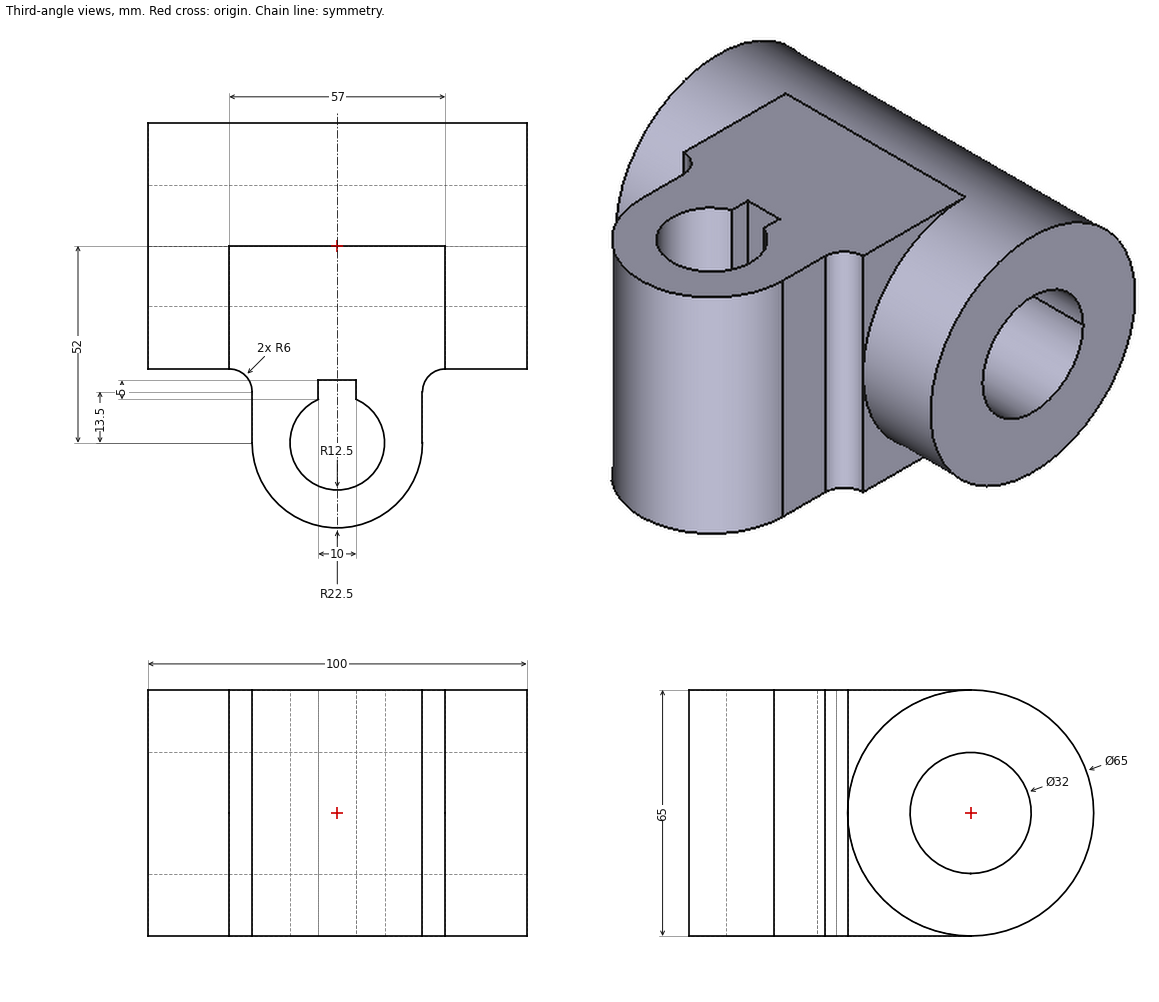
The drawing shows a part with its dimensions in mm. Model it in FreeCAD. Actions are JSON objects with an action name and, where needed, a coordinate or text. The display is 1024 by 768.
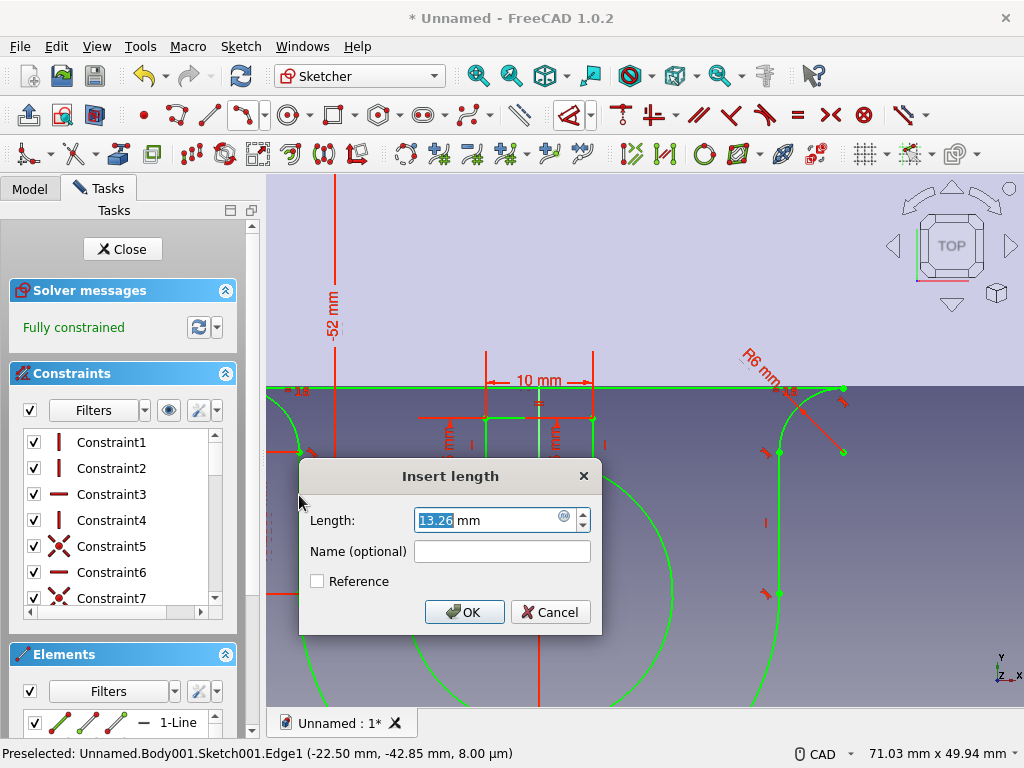
{"action": "type", "text": "13.5"}
{"action": "key", "text": "Return"}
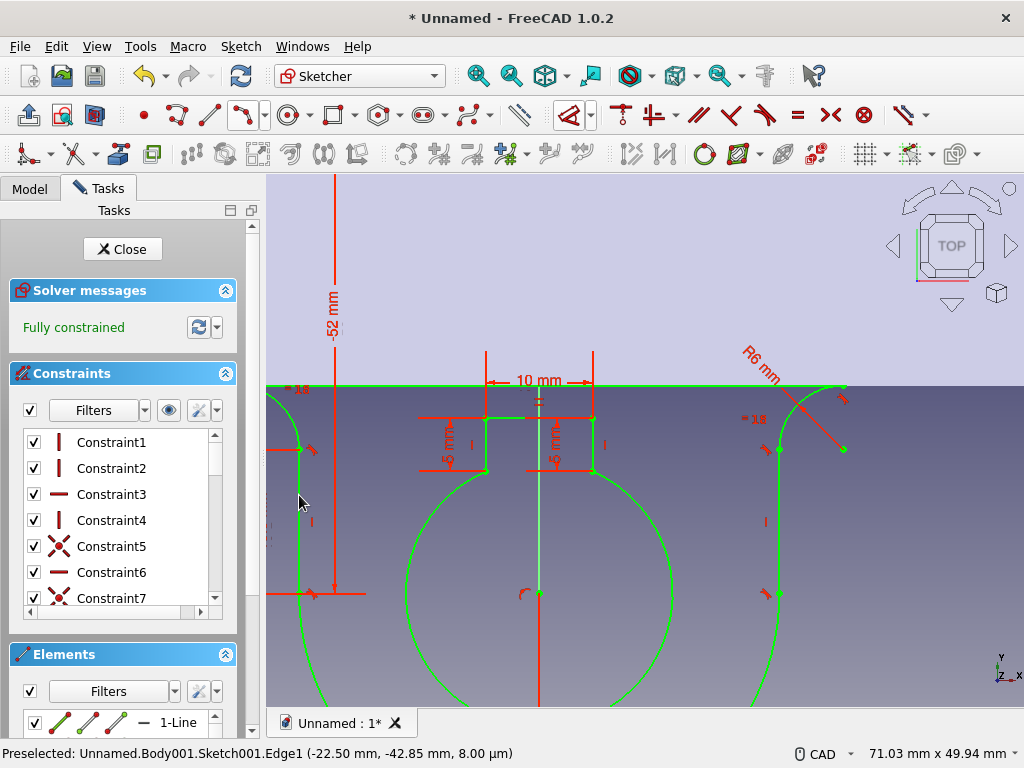
{"action": "left_click", "coordinate": [123, 249]}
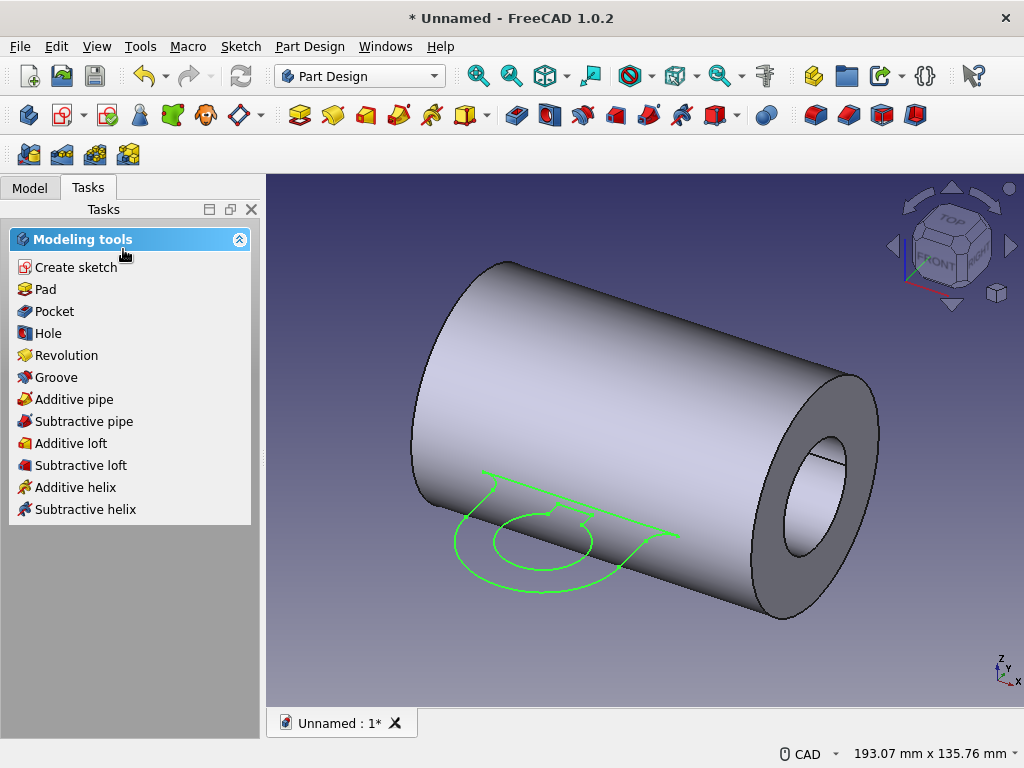
{"action": "left_click", "coordinate": [300, 116]}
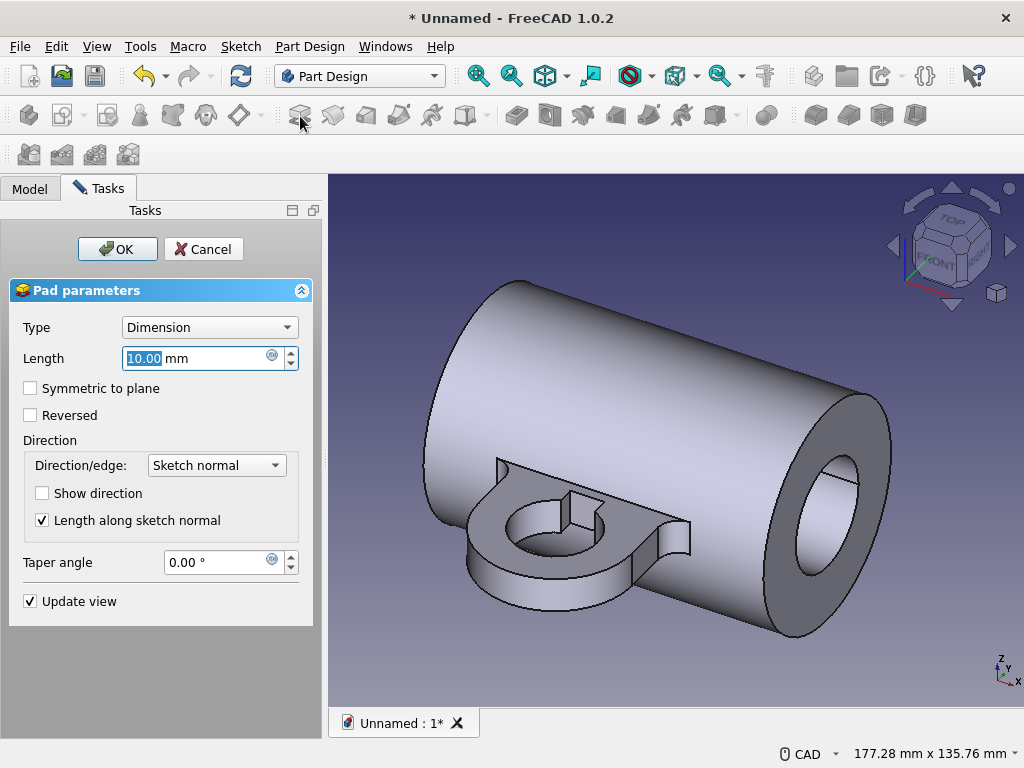
{"action": "type", "text": "65"}
{"action": "key", "text": "Tab"}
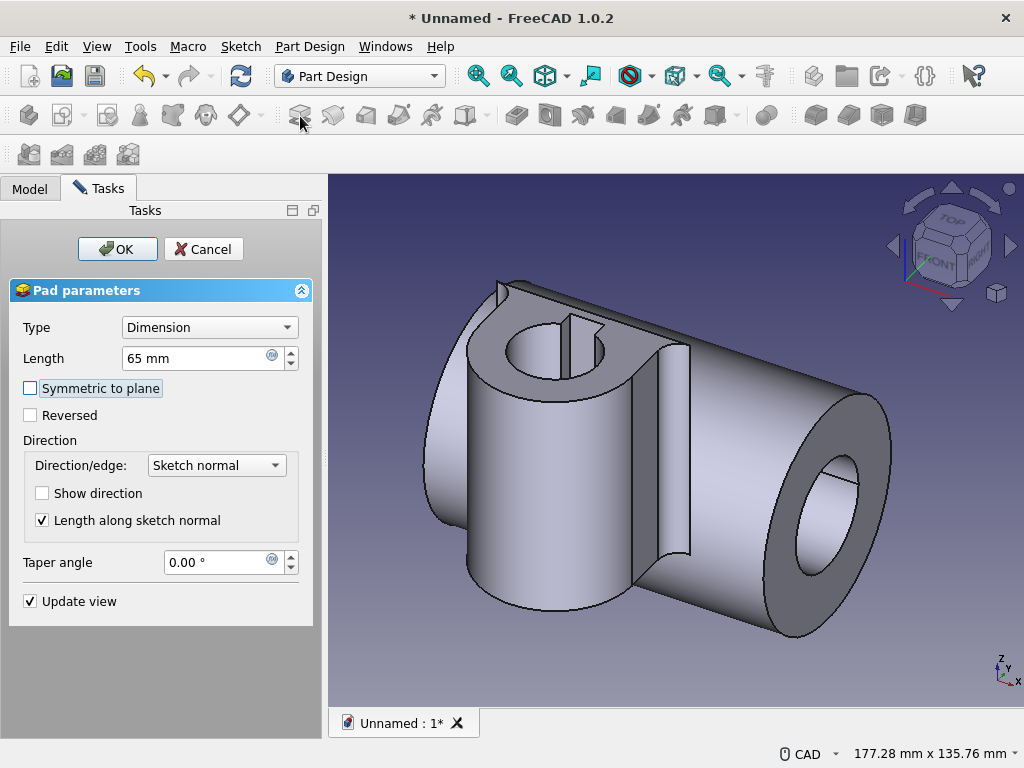
{"action": "left_click", "coordinate": [31, 388]}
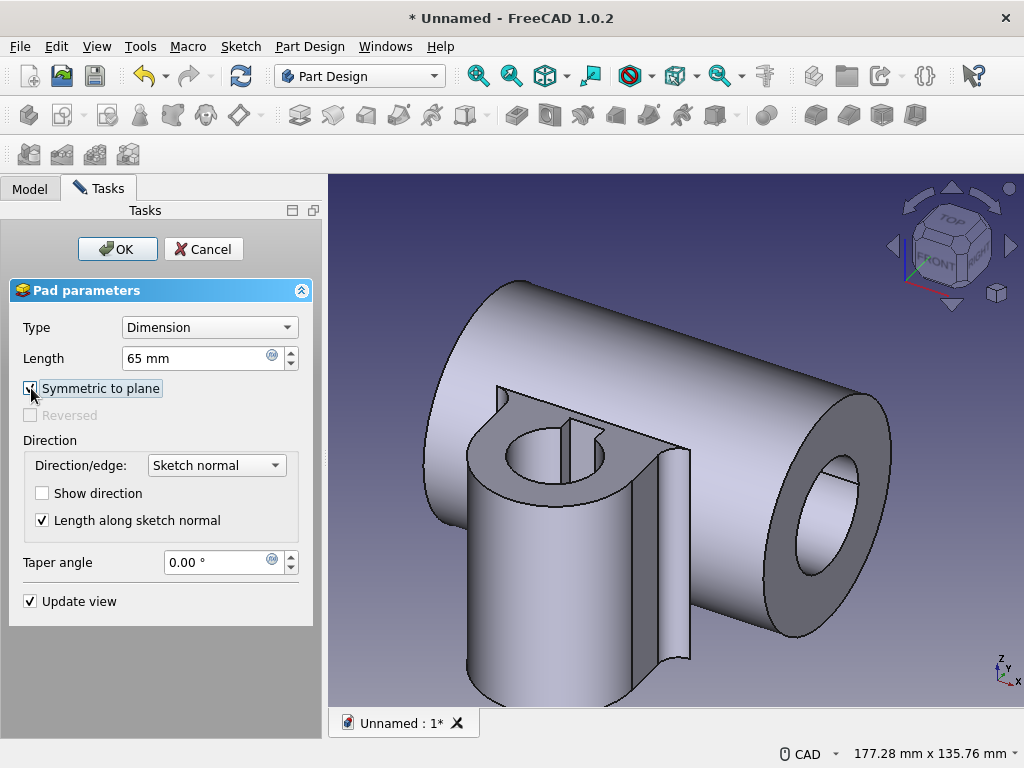
{"action": "left_click", "coordinate": [118, 249]}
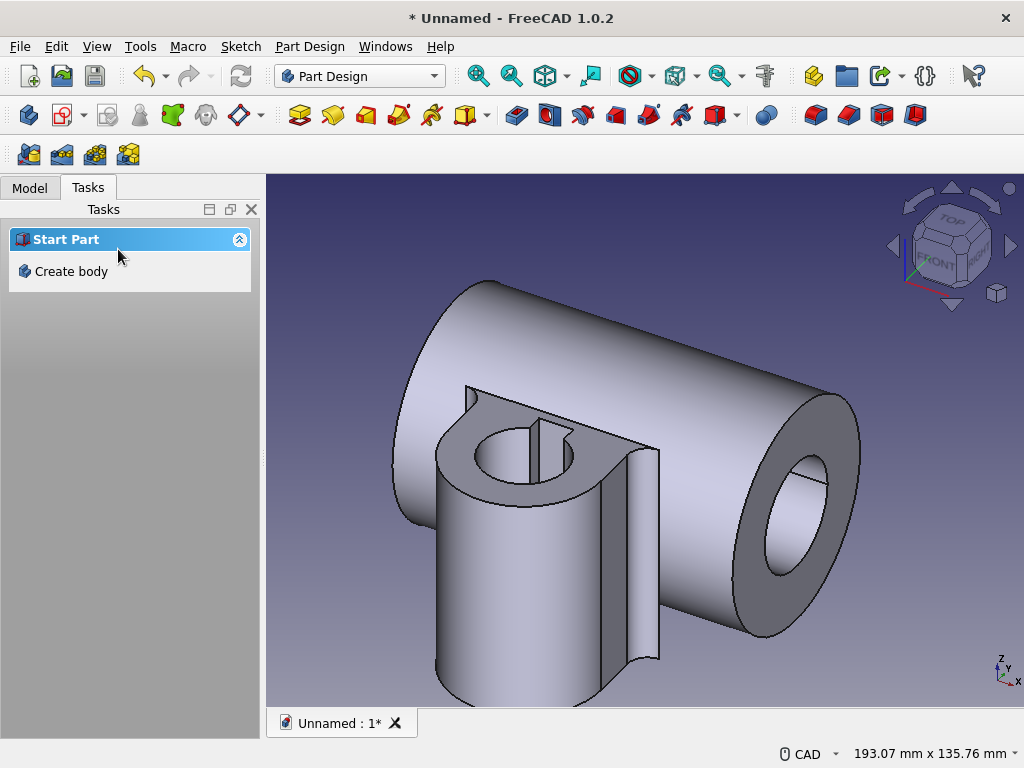
{"action": "key", "text": "v f"}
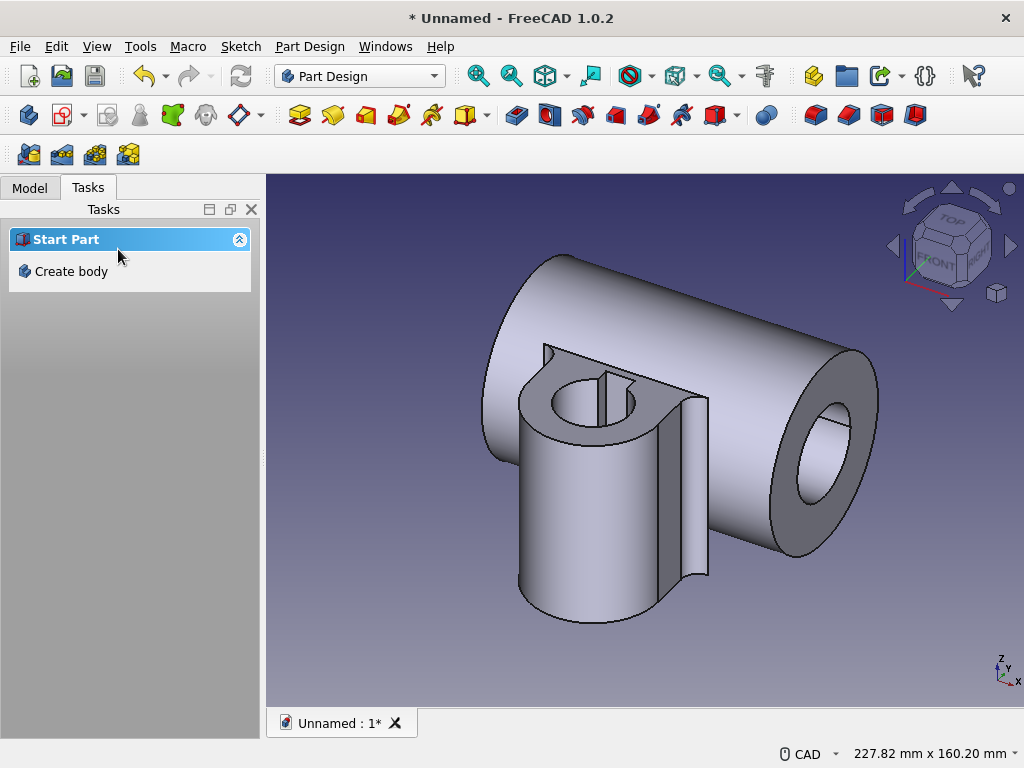
{"action": "left_click", "coordinate": [30, 188]}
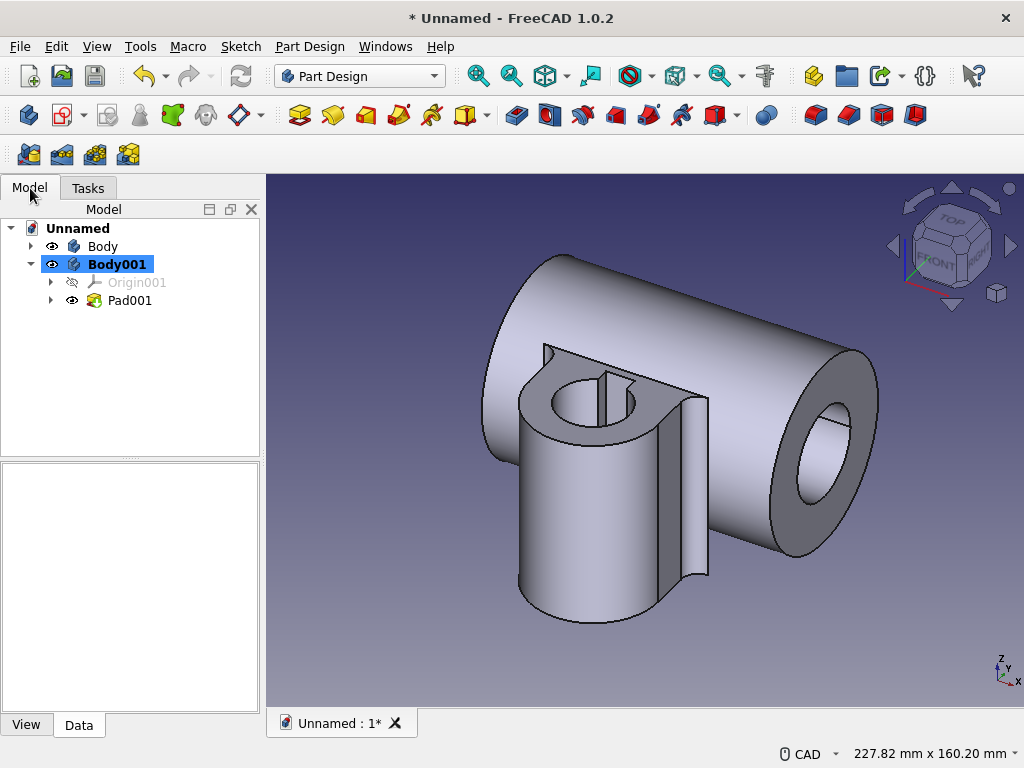
{"action": "double_click", "coordinate": [97, 246]}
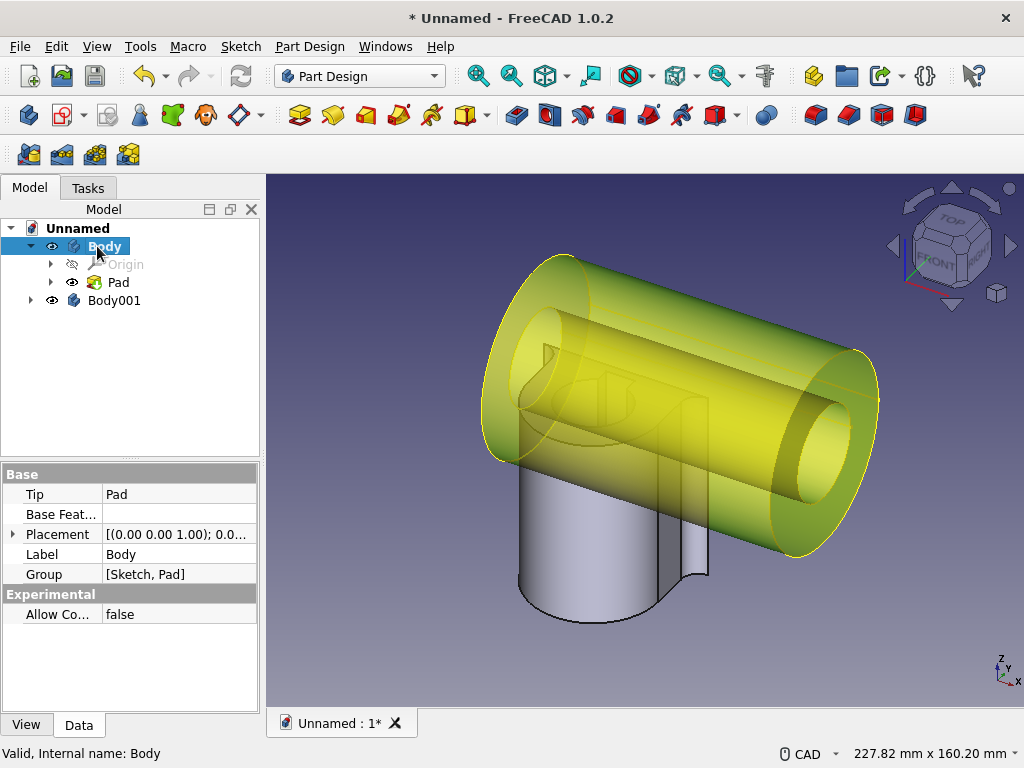
{"action": "left_click", "coordinate": [97, 246]}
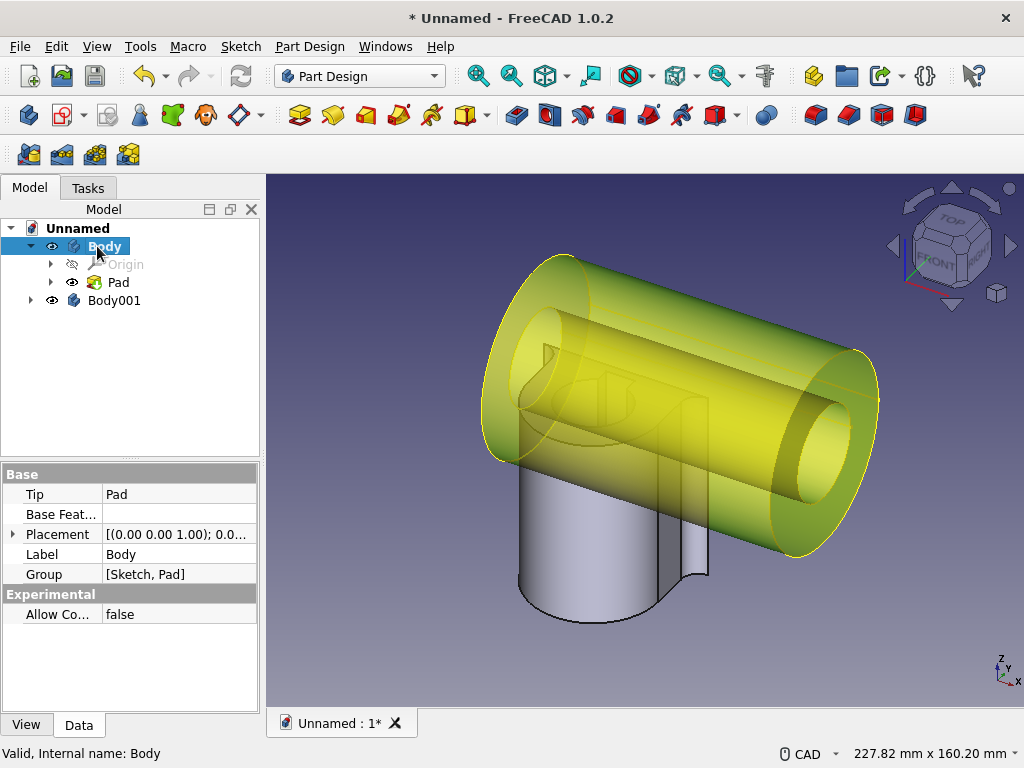
{"action": "left_click", "coordinate": [148, 614]}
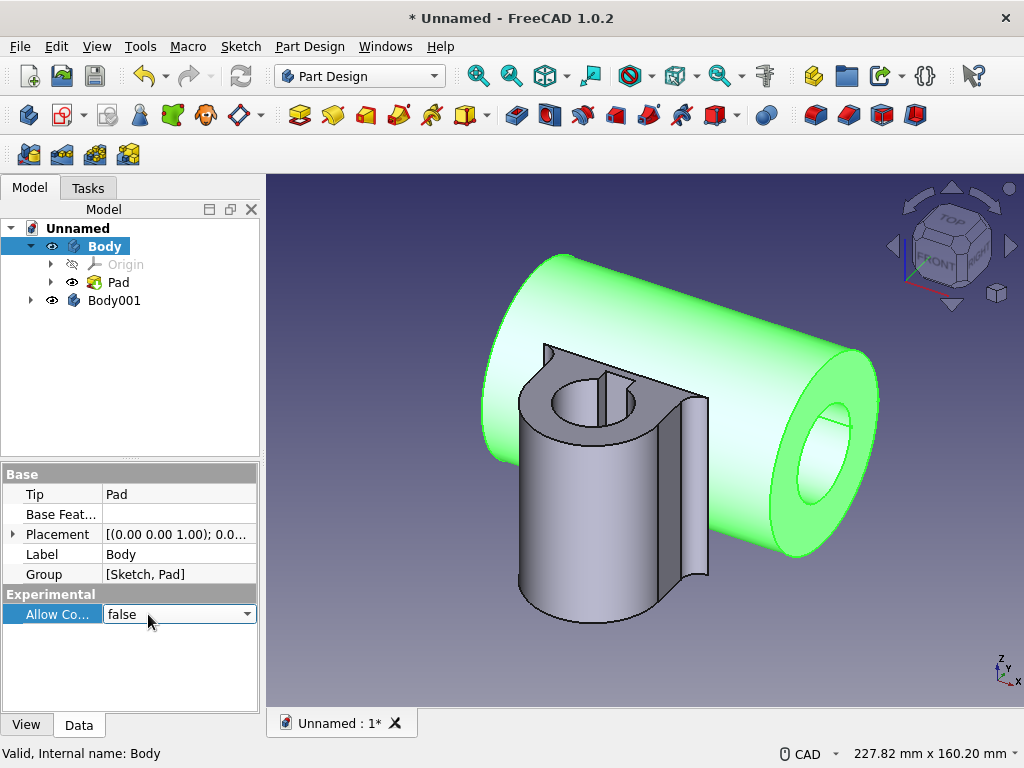
{"action": "left_click", "coordinate": [148, 614]}